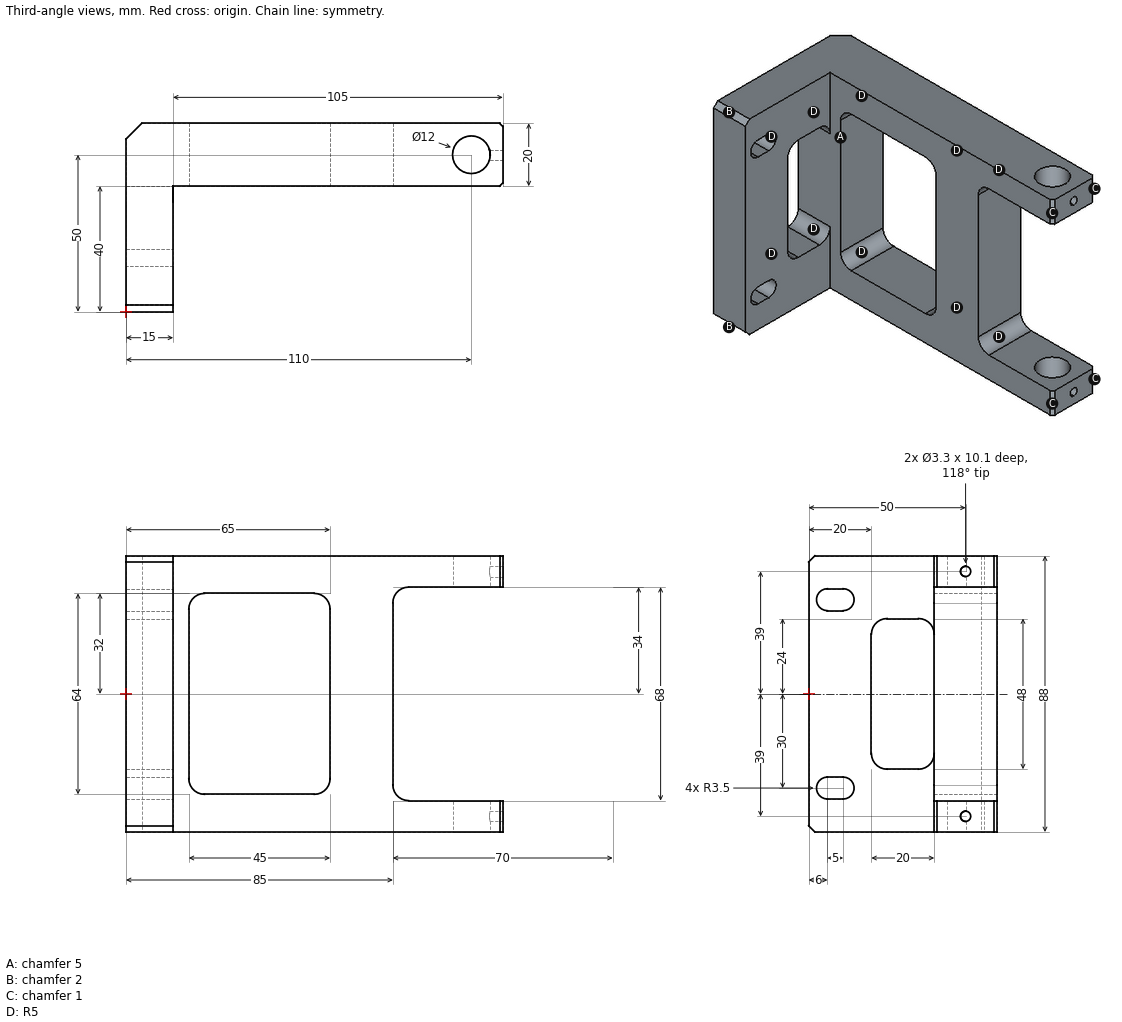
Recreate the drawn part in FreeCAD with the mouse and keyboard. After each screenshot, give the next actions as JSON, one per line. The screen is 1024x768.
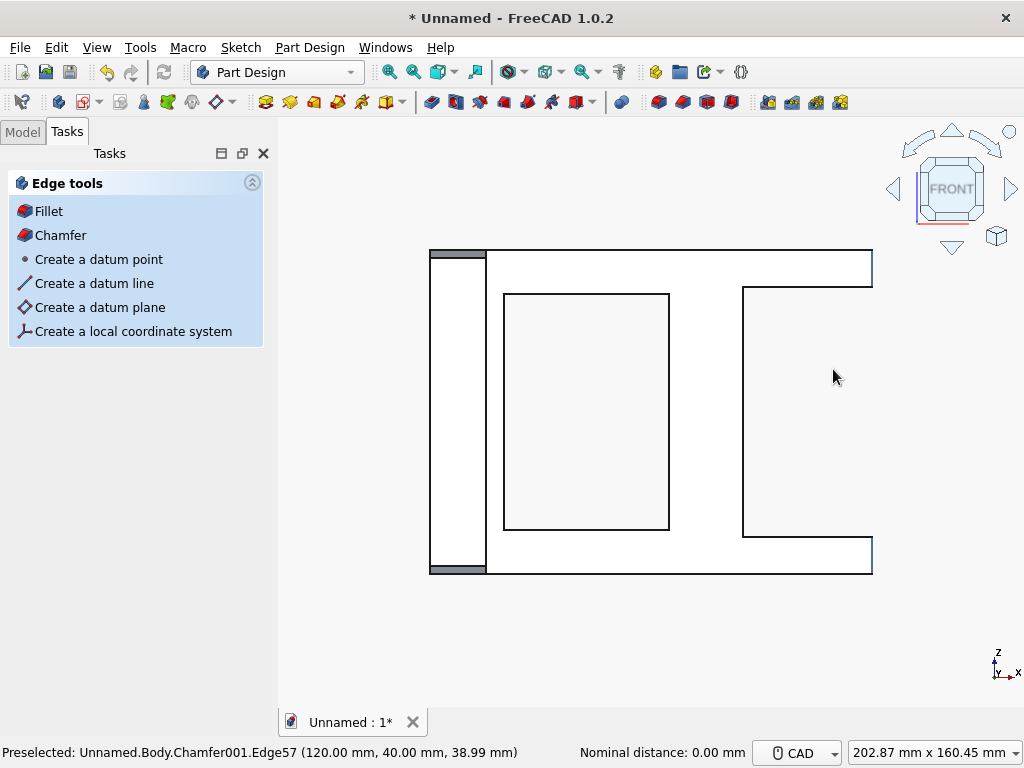
{"action": "key", "text": "3"}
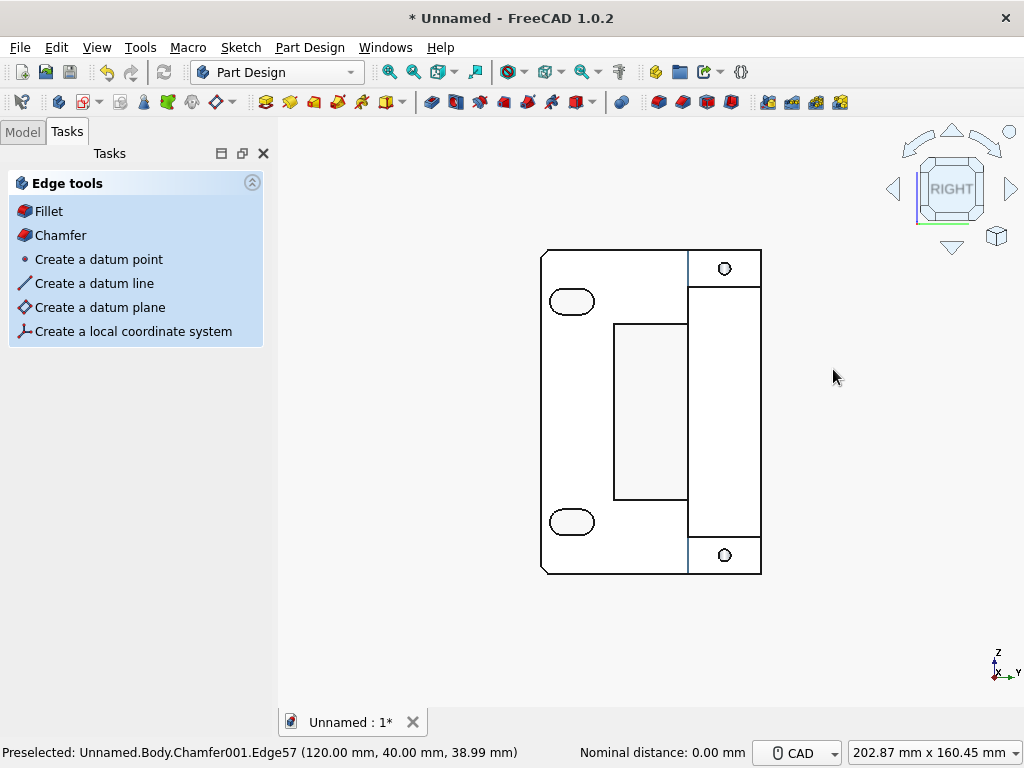
{"action": "left_click", "coordinate": [761, 268], "text": "ctrl"}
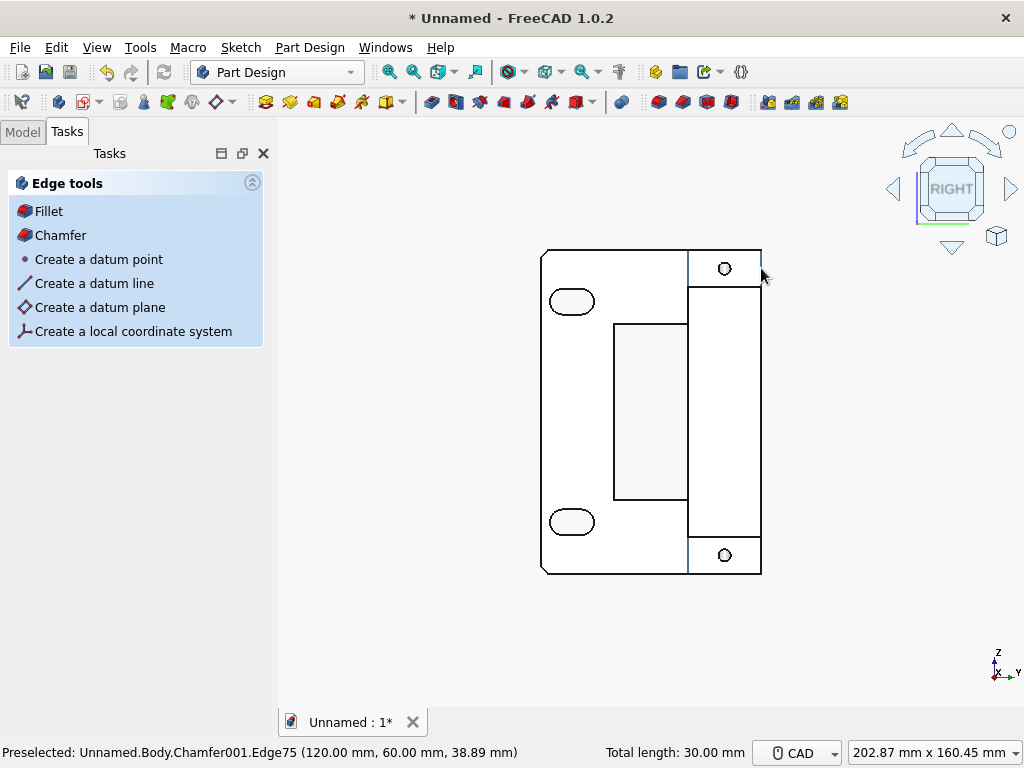
{"action": "left_click", "coordinate": [761, 554], "text": "ctrl"}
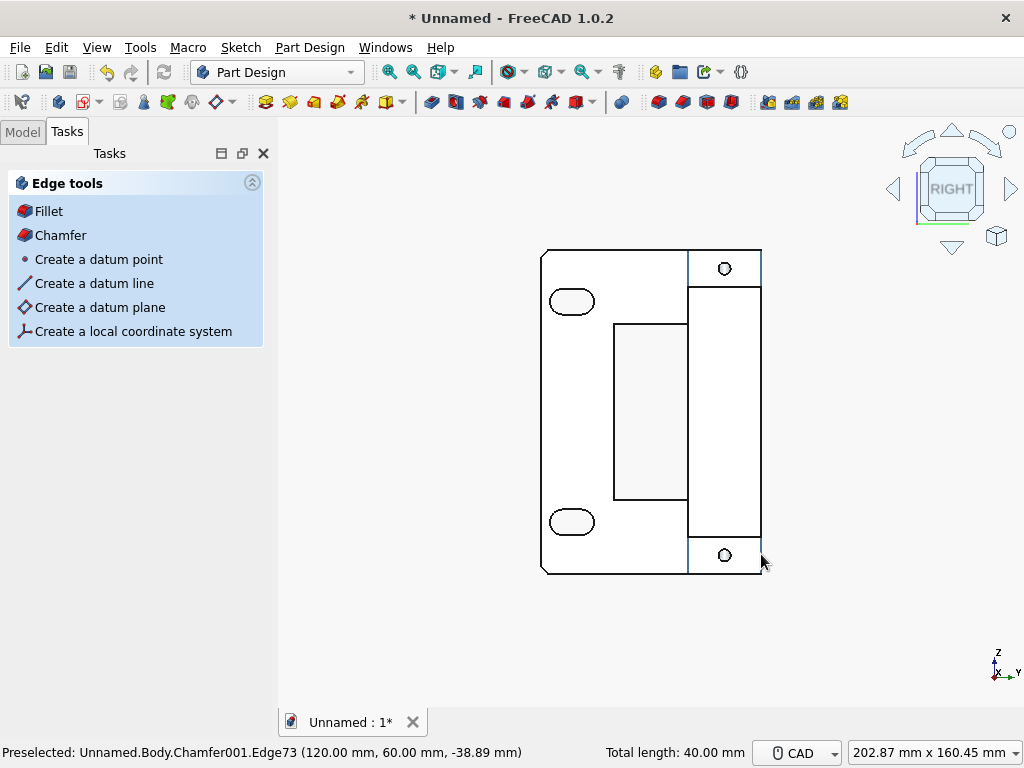
{"action": "left_click", "coordinate": [684, 102]}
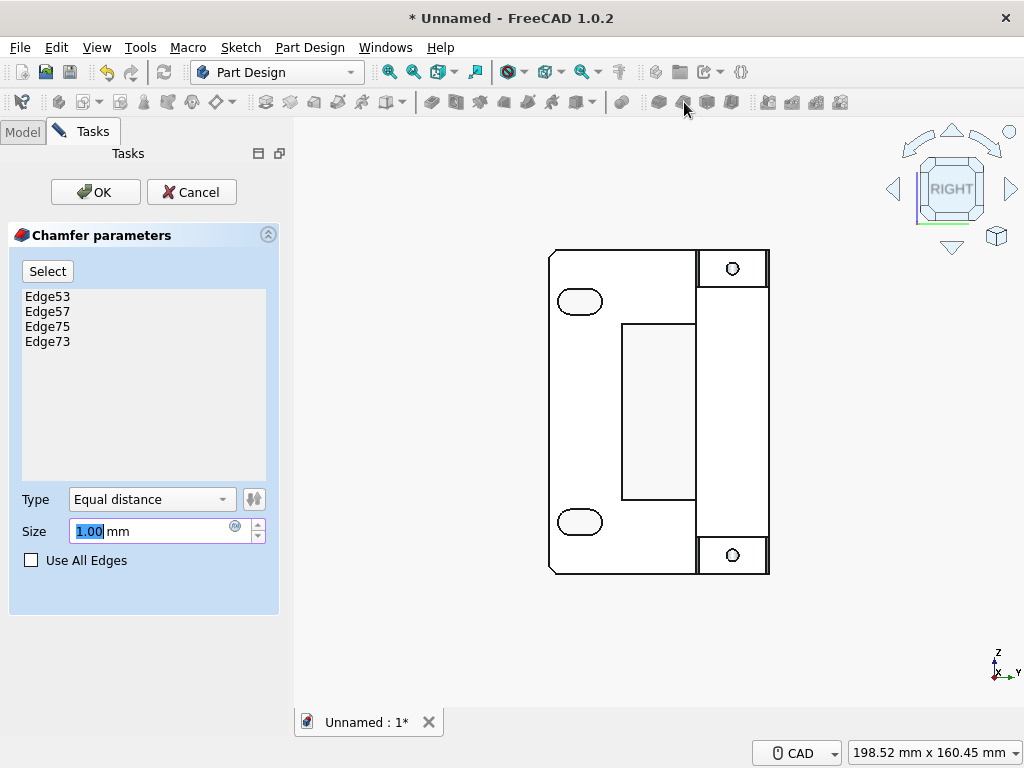
{"action": "type", "text": "1"}
{"action": "key", "text": "Tab"}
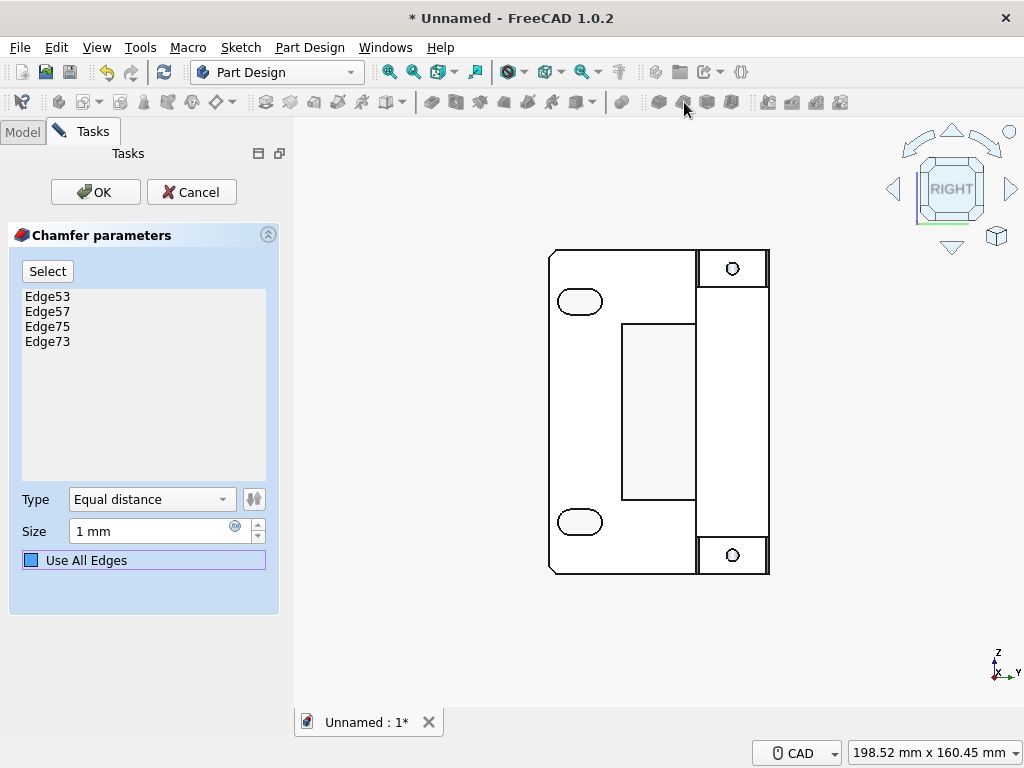
{"action": "left_click", "coordinate": [96, 192]}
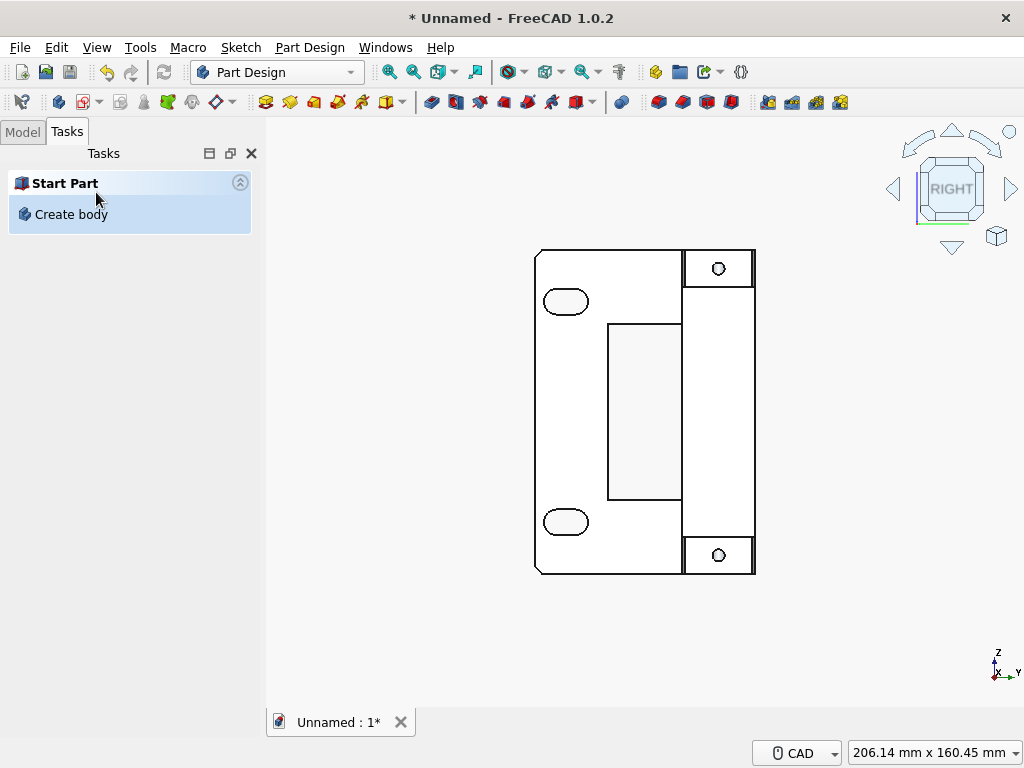
{"action": "key", "text": "0"}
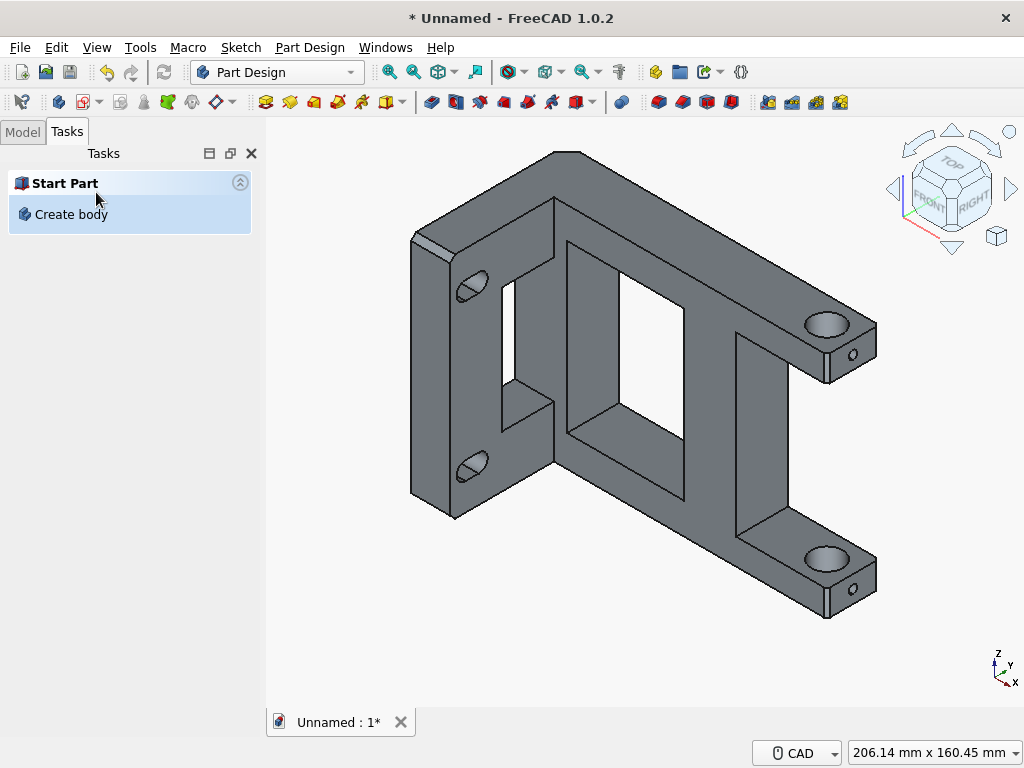
{"action": "key", "text": "2"}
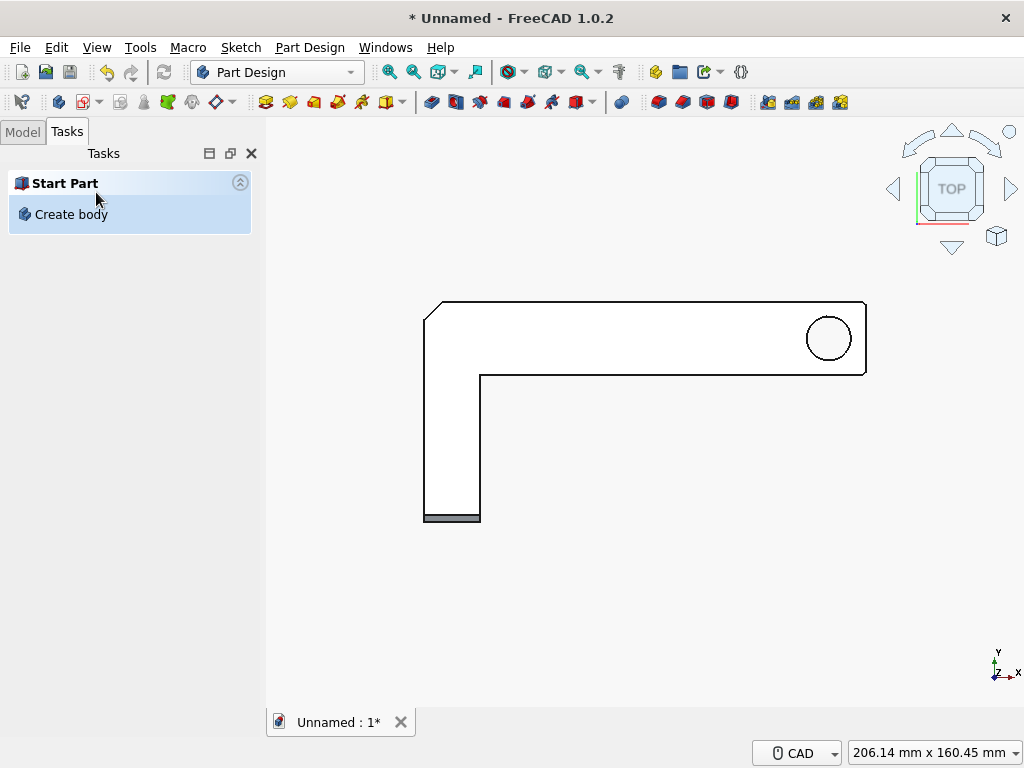
{"action": "key", "text": "1"}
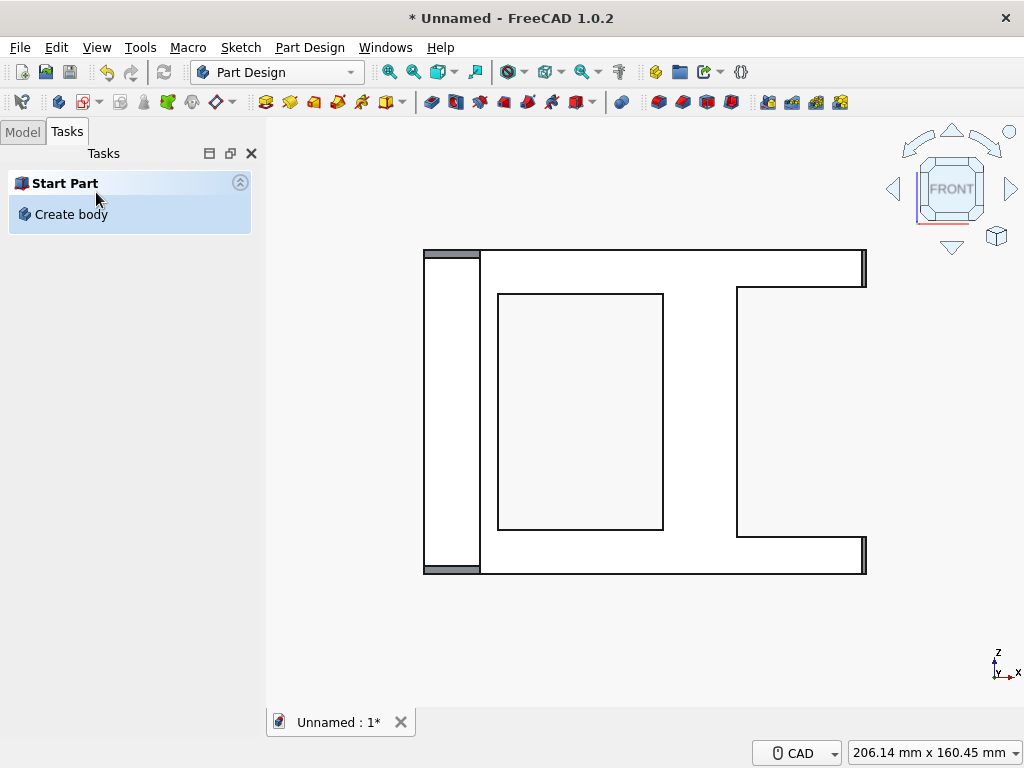
{"action": "key", "text": "3"}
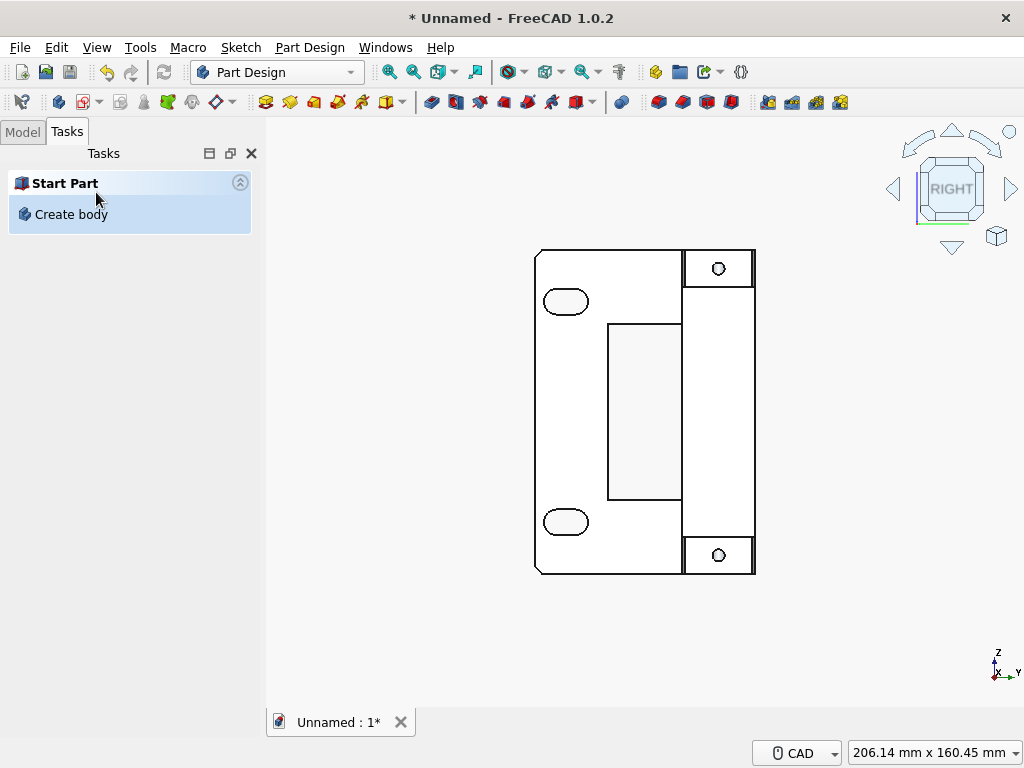
{"action": "key", "text": "5"}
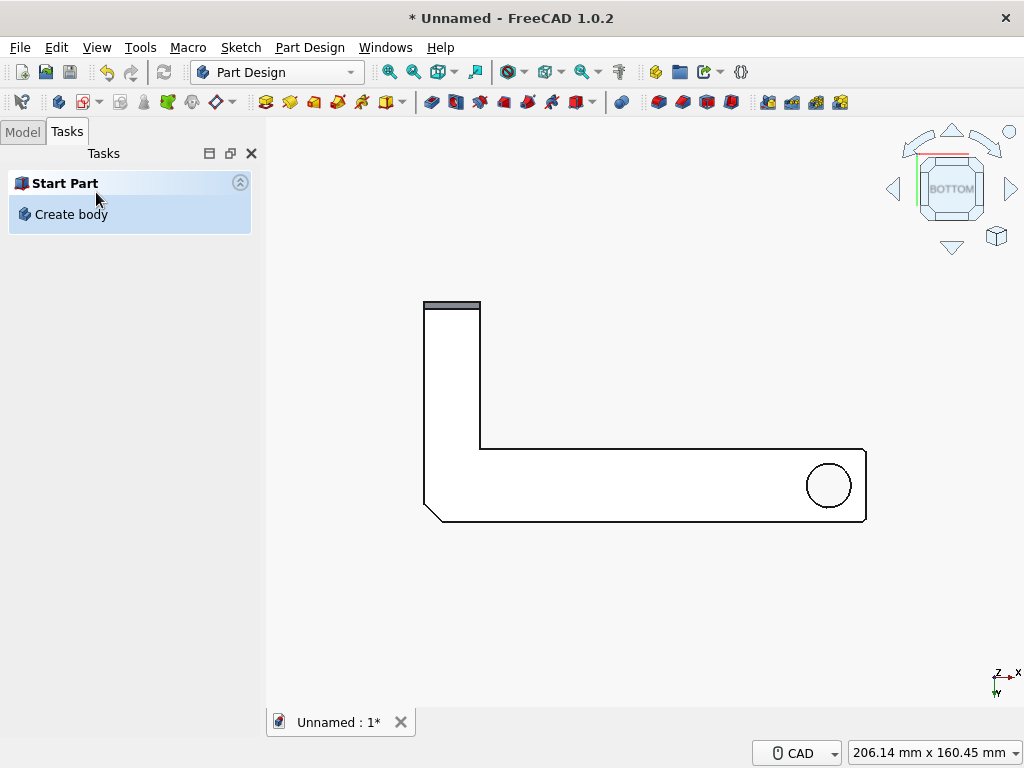
{"action": "key", "text": "4"}